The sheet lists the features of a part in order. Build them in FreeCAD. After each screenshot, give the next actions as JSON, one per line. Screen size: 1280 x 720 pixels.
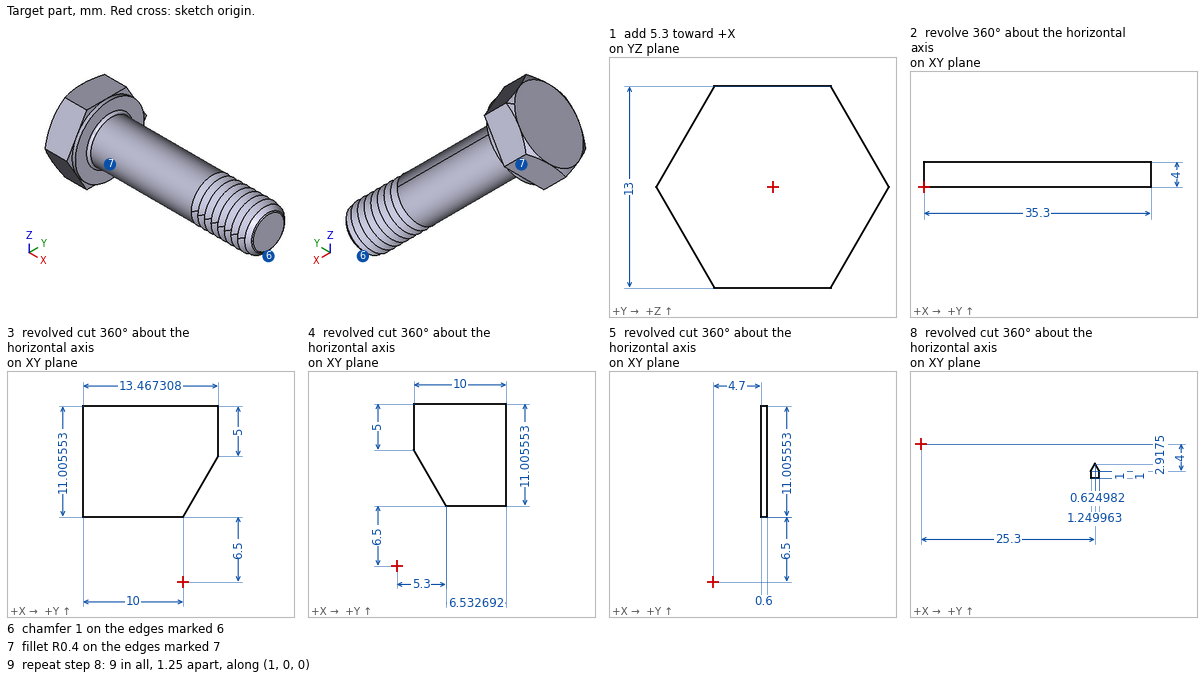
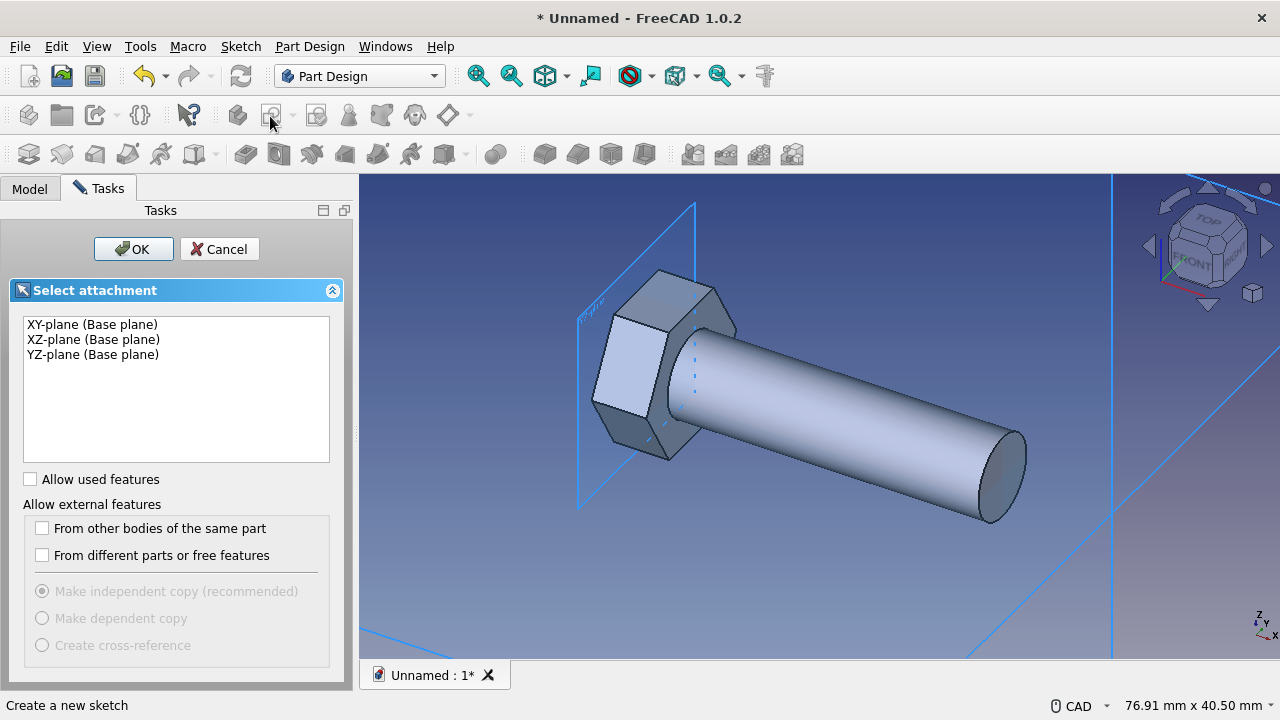
{"action": "left_click", "coordinate": [84, 324]}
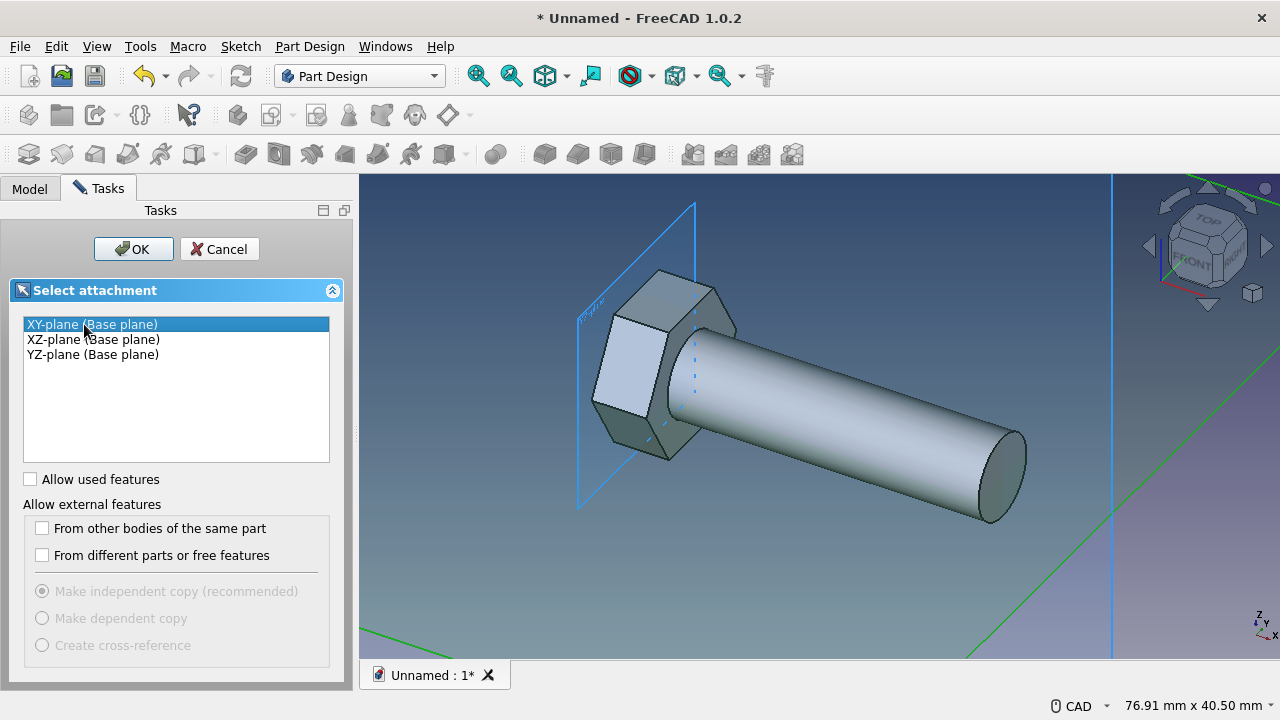
{"action": "left_click", "coordinate": [134, 249]}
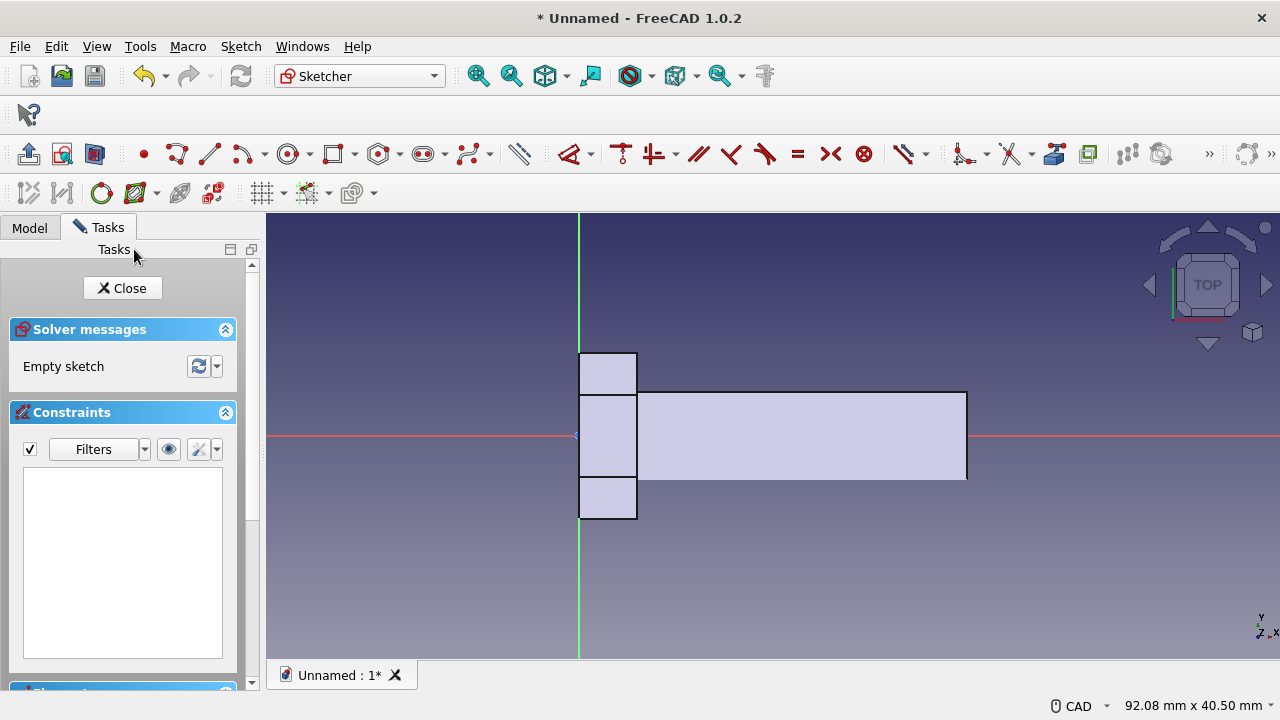
{"action": "left_click", "coordinate": [95, 154]}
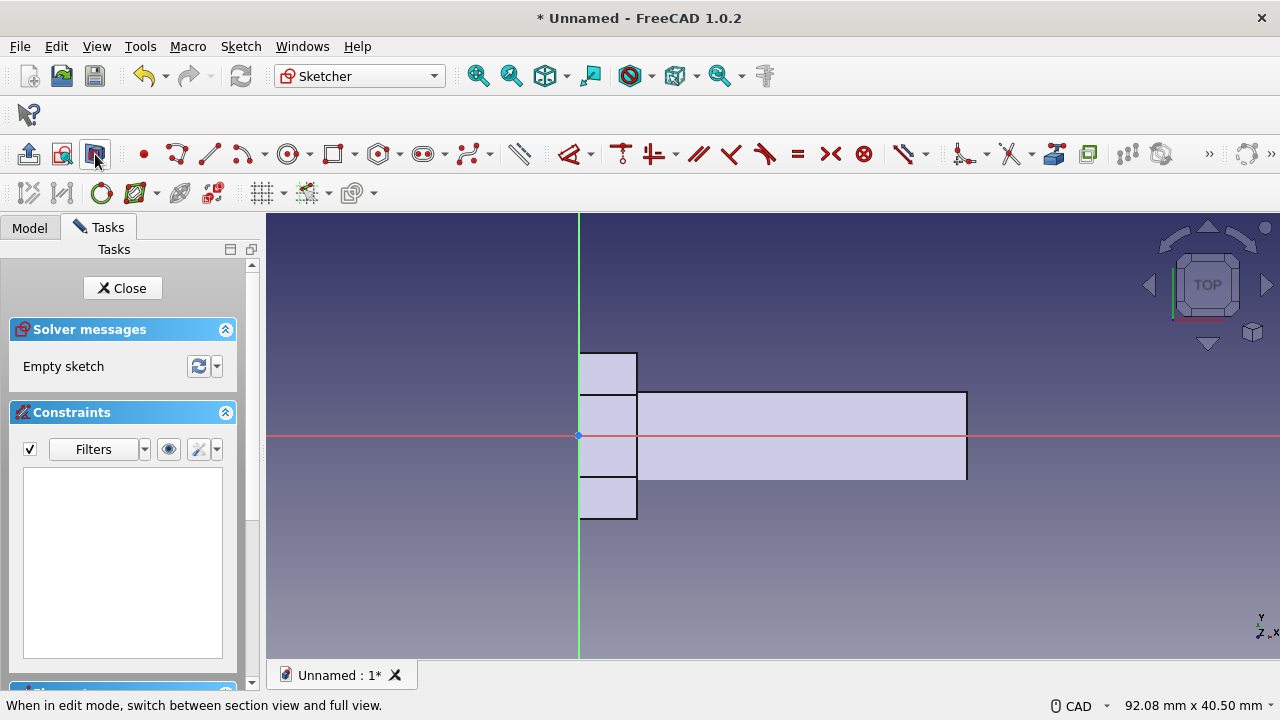
{"action": "scroll", "coordinate": [1115, 631], "scroll_direction": "down", "scroll_amount": 1}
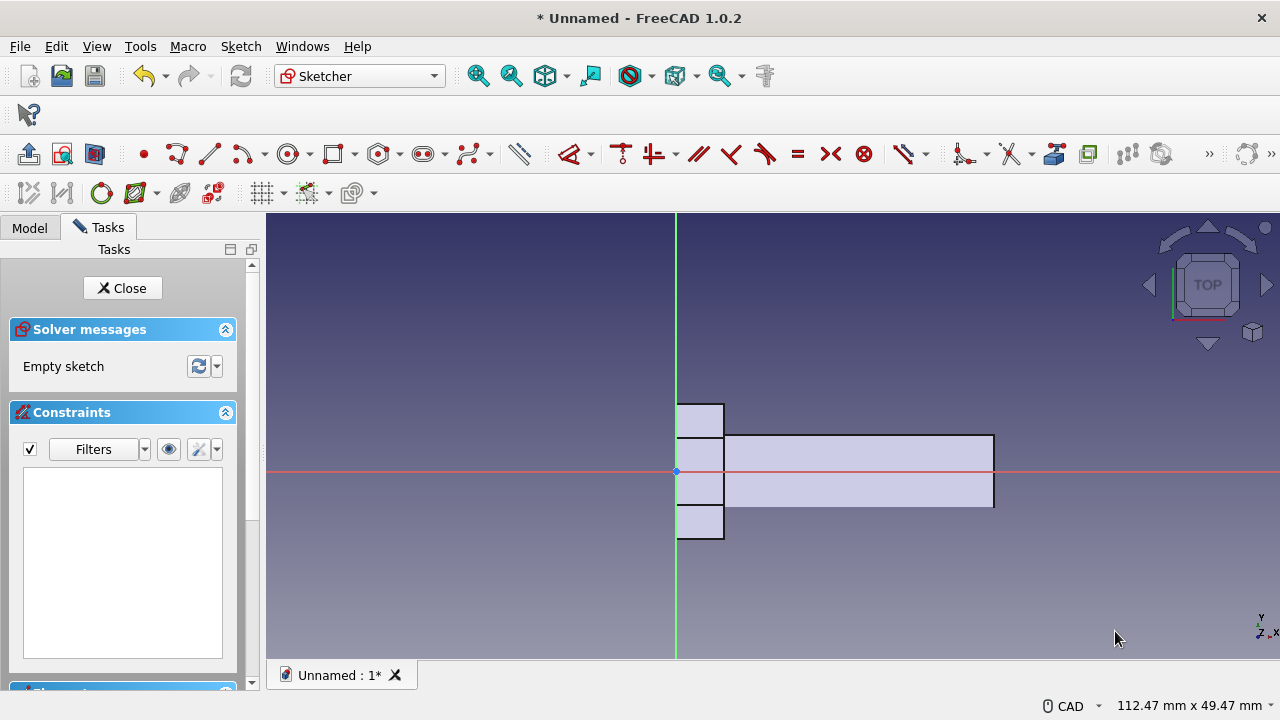
{"action": "scroll", "coordinate": [576, 340], "scroll_direction": "up", "scroll_amount": 3}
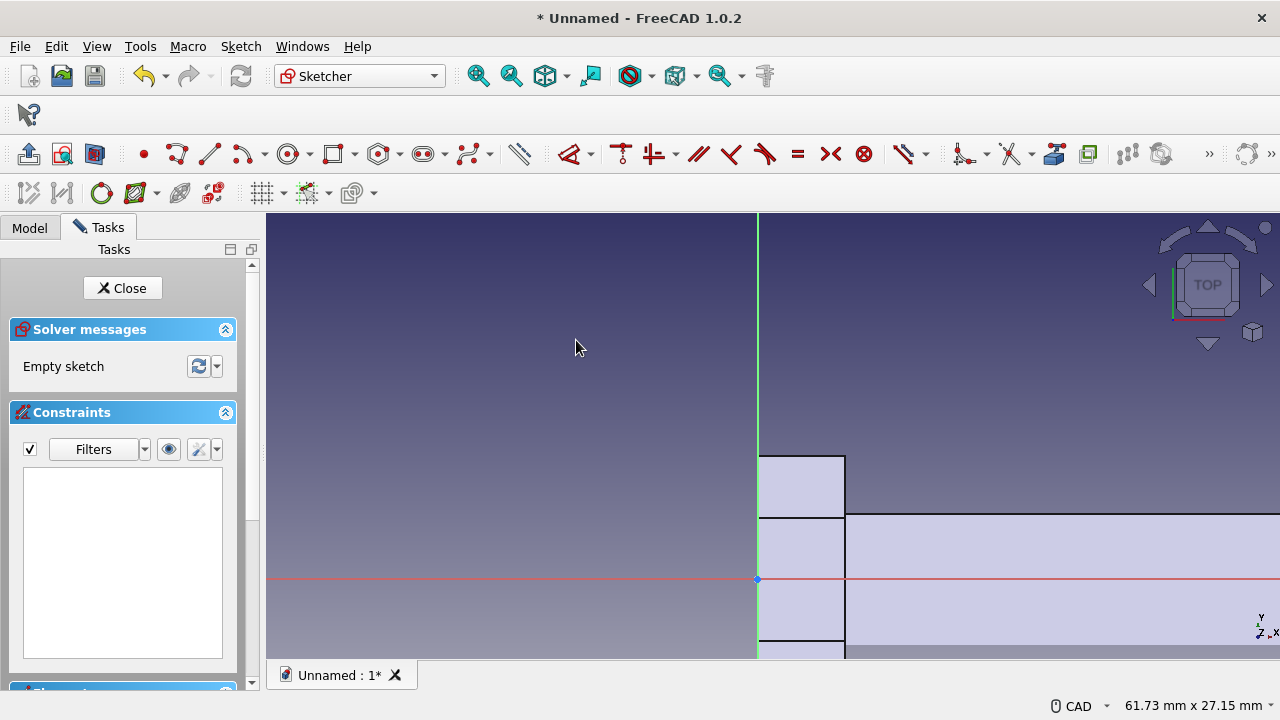
{"action": "left_click", "coordinate": [177, 154]}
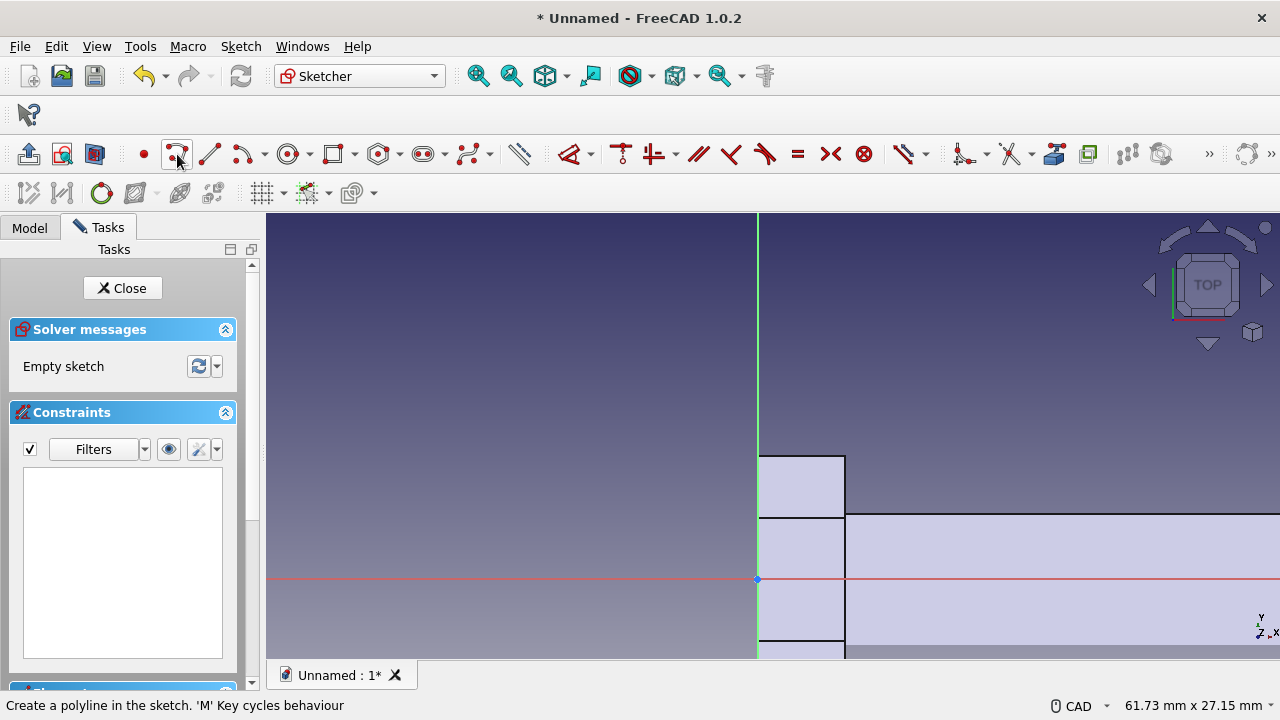
{"action": "left_click", "coordinate": [758, 473]}
{"action": "left_click", "coordinate": [815, 374]}
{"action": "left_click", "coordinate": [815, 292]}
{"action": "left_click", "coordinate": [594, 292]}
{"action": "left_click", "coordinate": [594, 473]}
{"action": "left_click", "coordinate": [758, 474]}
{"action": "key", "text": "Escape"}
{"action": "key", "text": "Escape"}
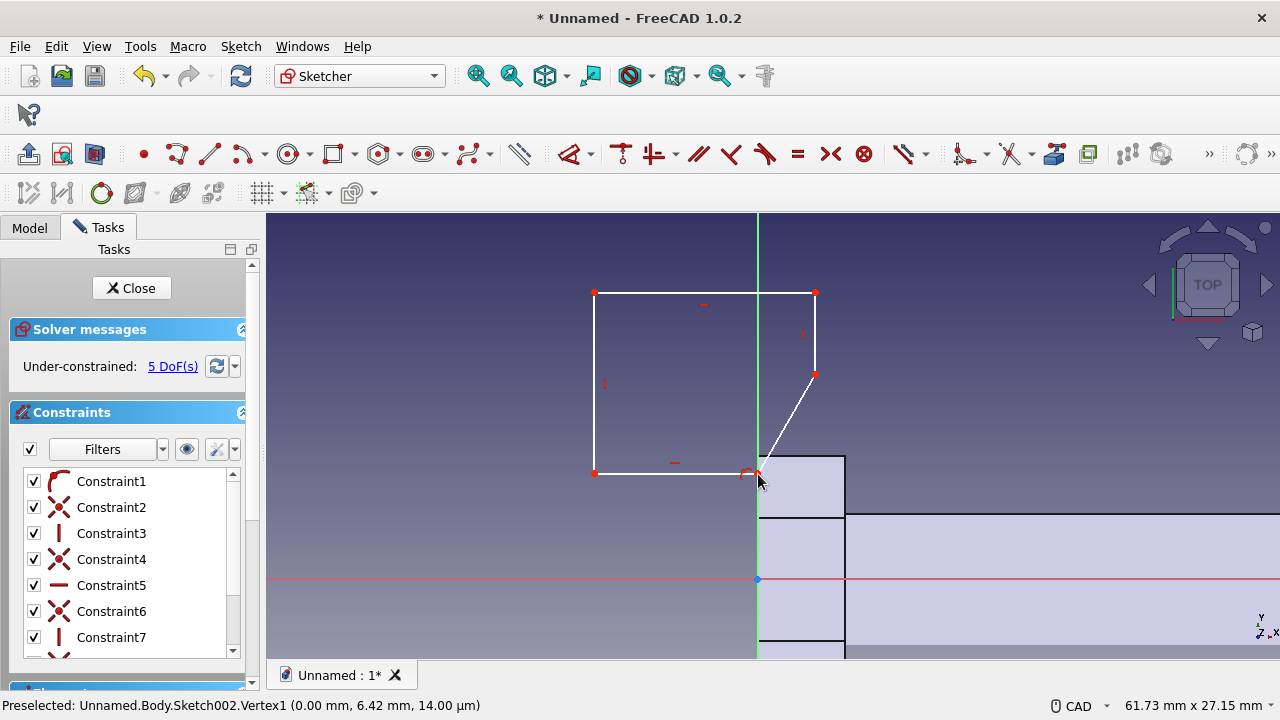
{"action": "left_click", "coordinate": [568, 154]}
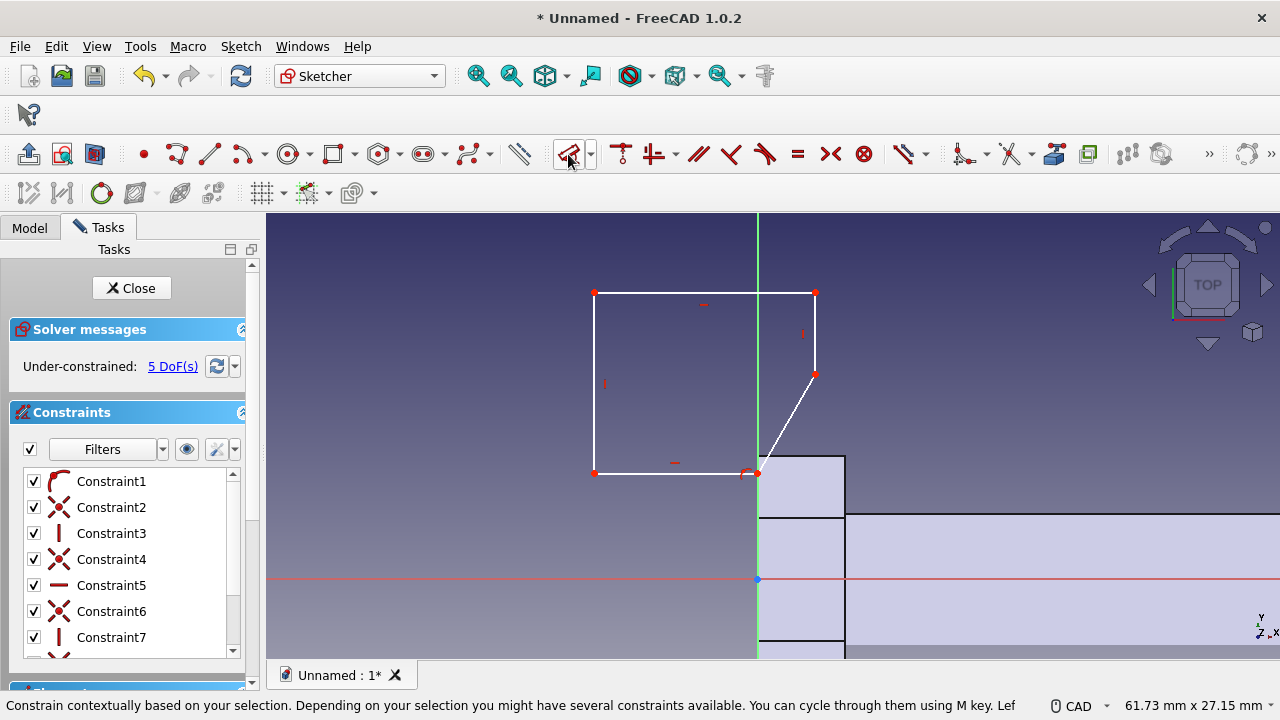
{"action": "left_click", "coordinate": [815, 350]}
{"action": "left_click", "coordinate": [849, 334]}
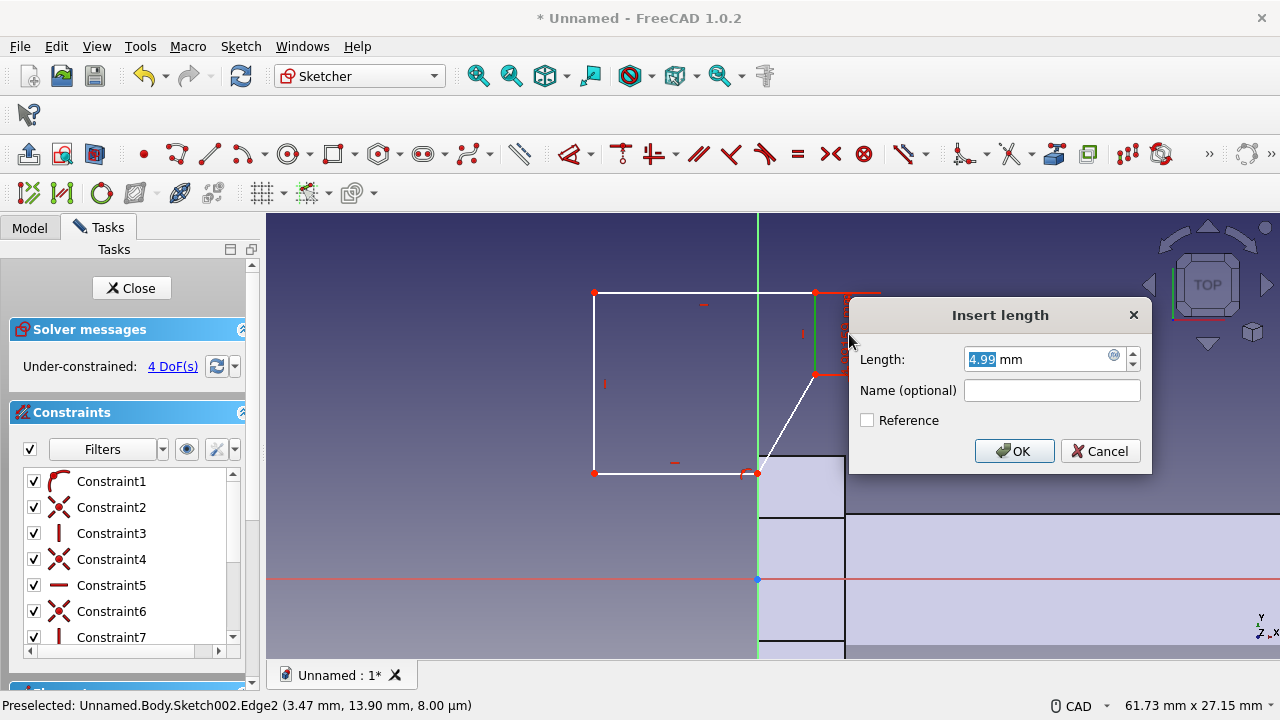
{"action": "type", "text": "5"}
{"action": "key", "text": "Return"}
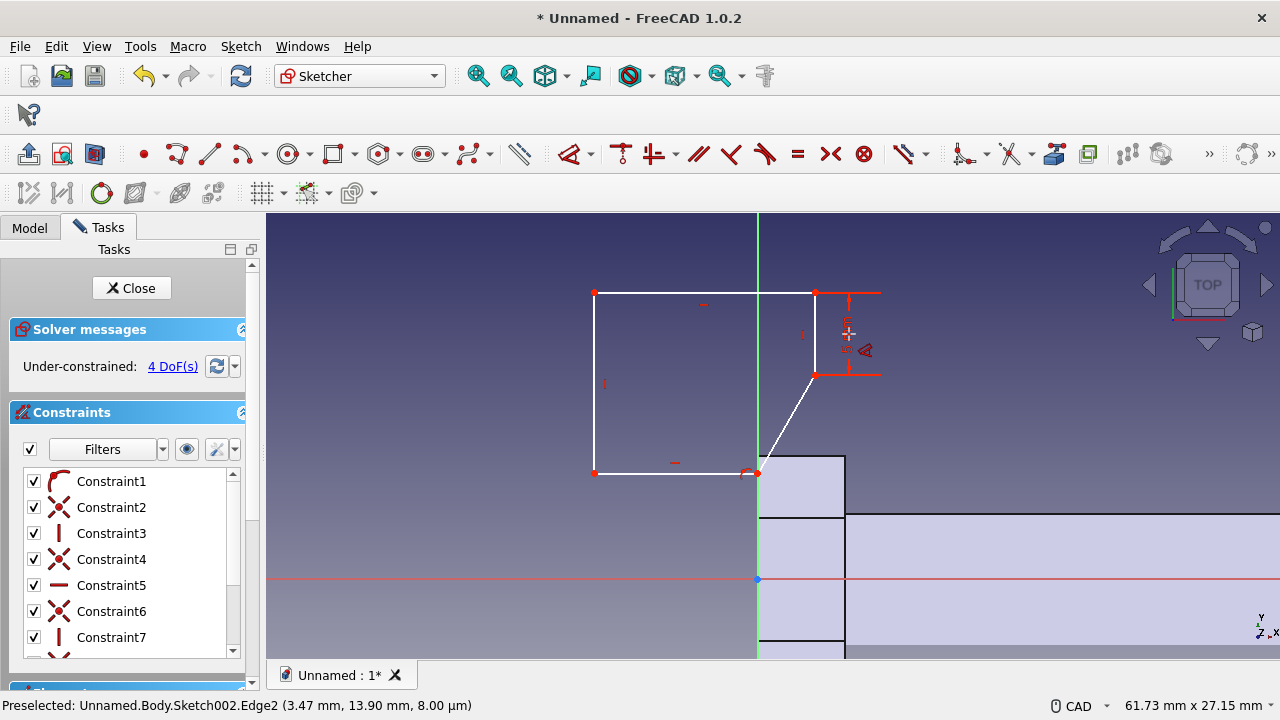
{"action": "left_click", "coordinate": [643, 474]}
{"action": "left_click", "coordinate": [676, 508]}